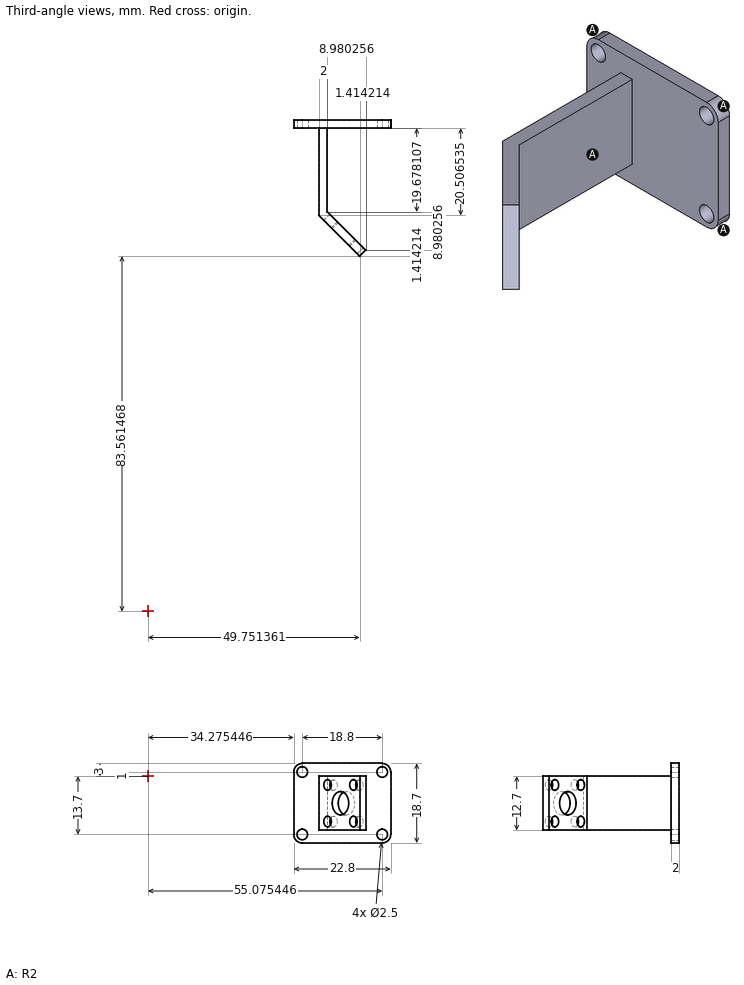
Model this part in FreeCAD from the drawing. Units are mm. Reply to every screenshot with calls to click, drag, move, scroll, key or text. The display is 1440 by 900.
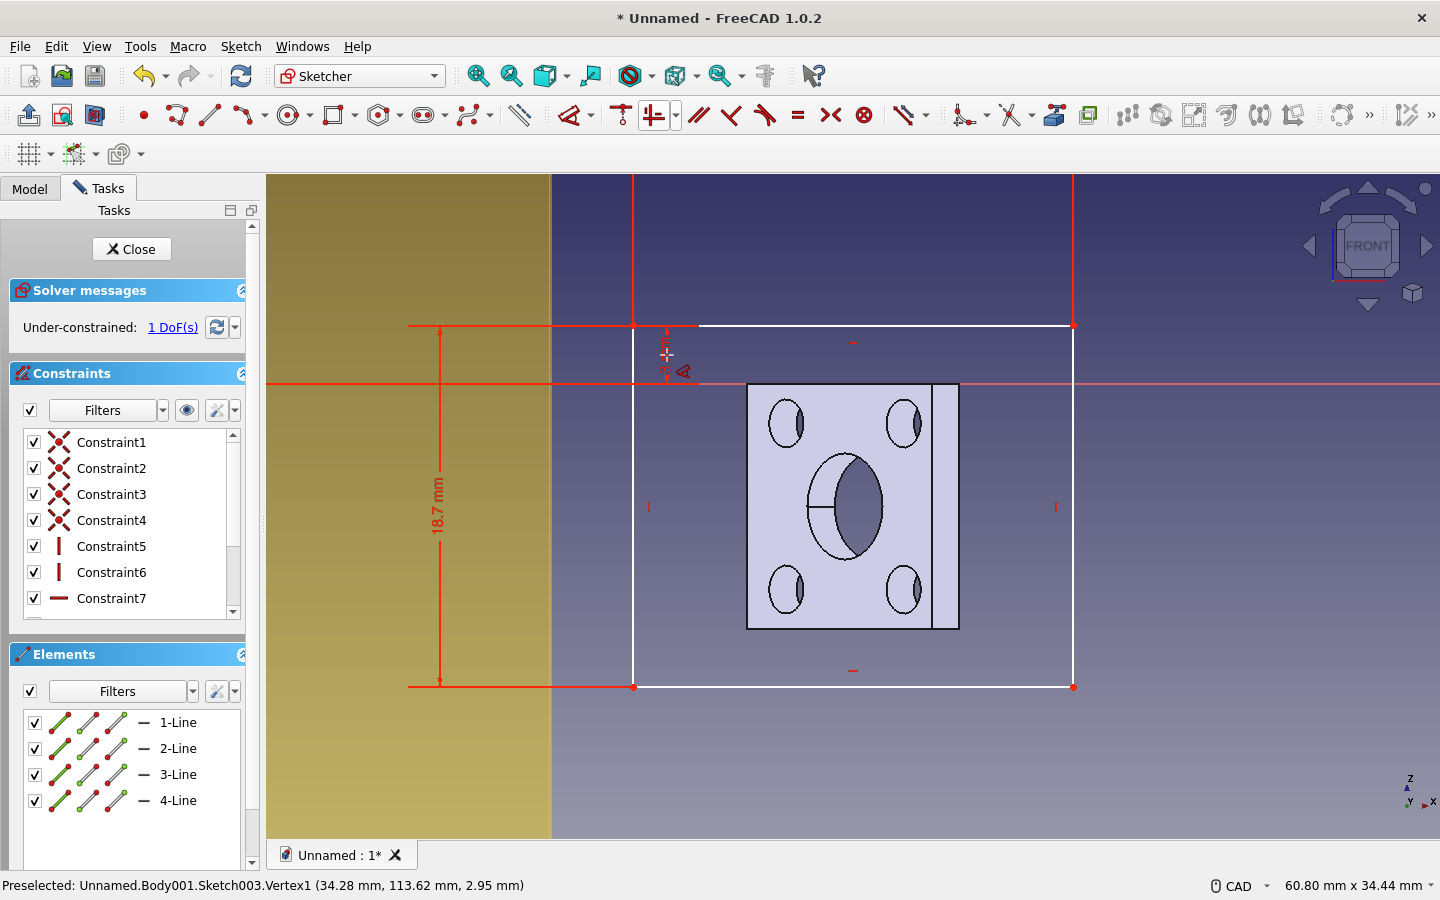
click(633, 326)
click(463, 292)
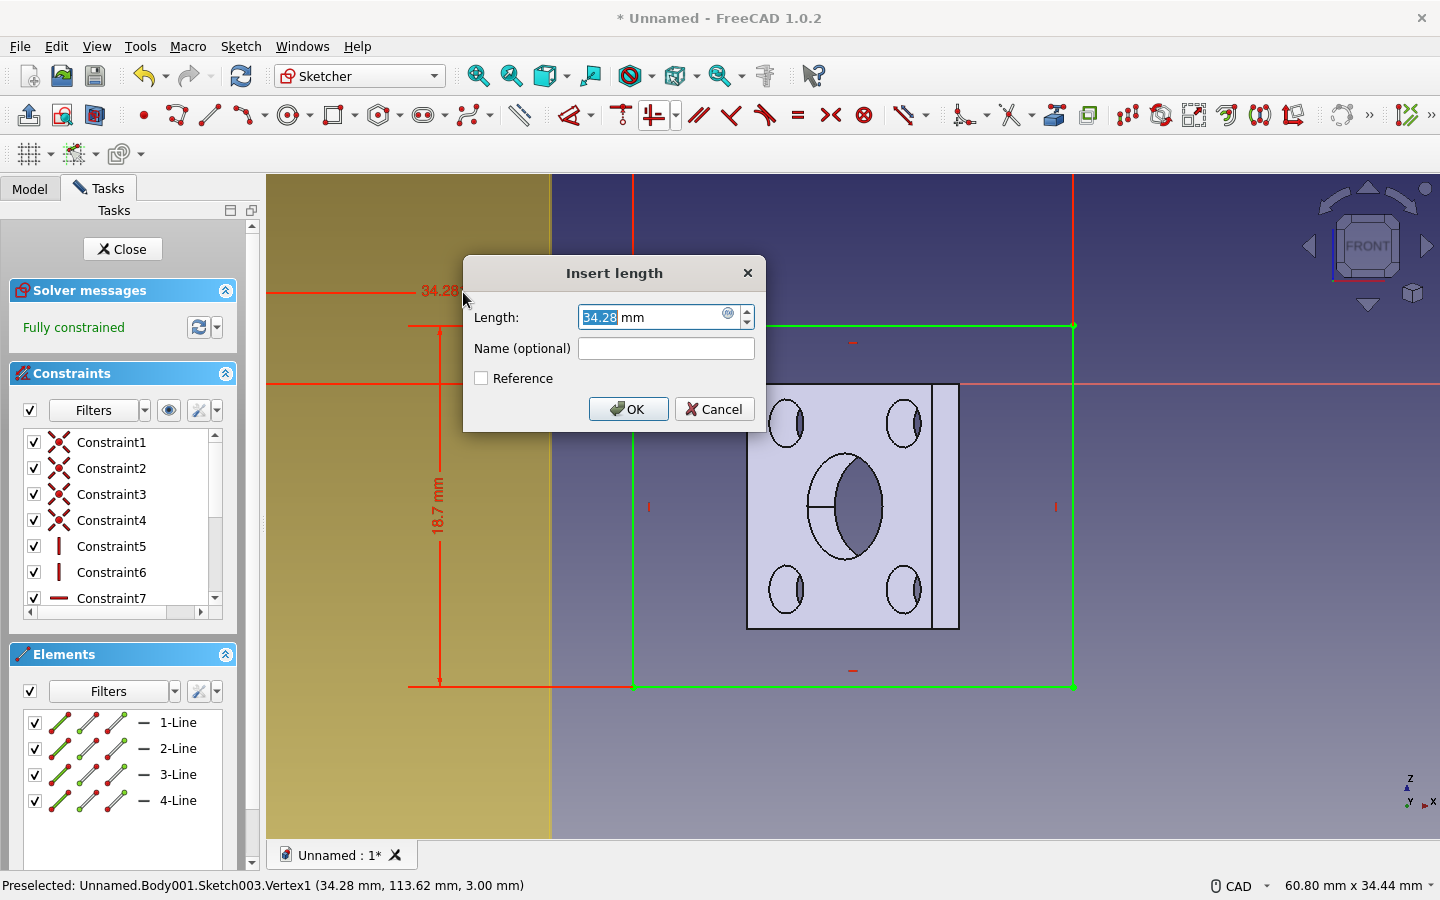
text(34.275446)
key(Return)
key(Escape)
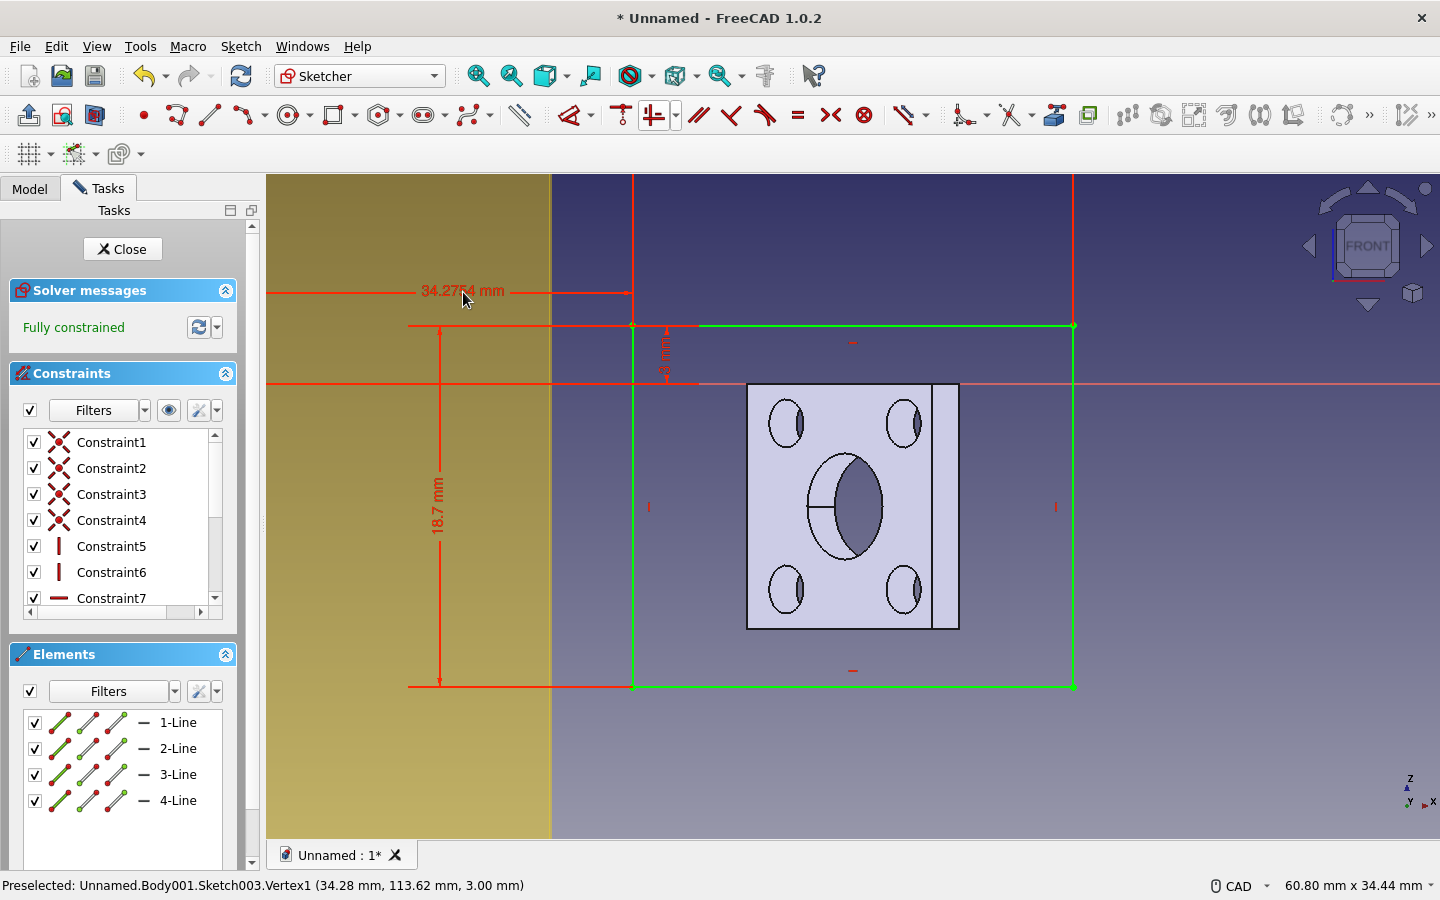
click(123, 249)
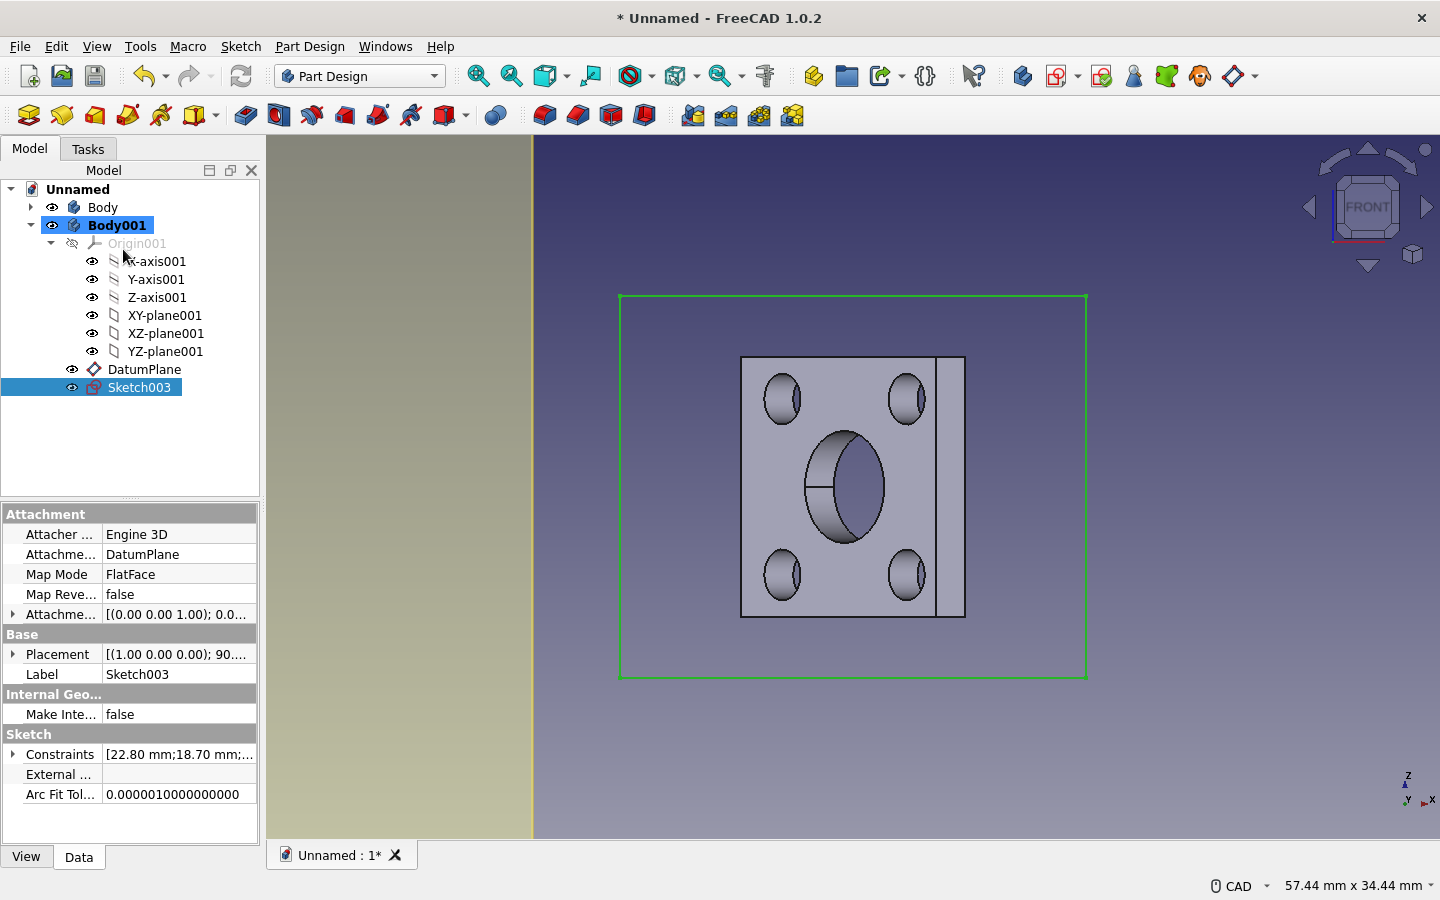
click(29, 116)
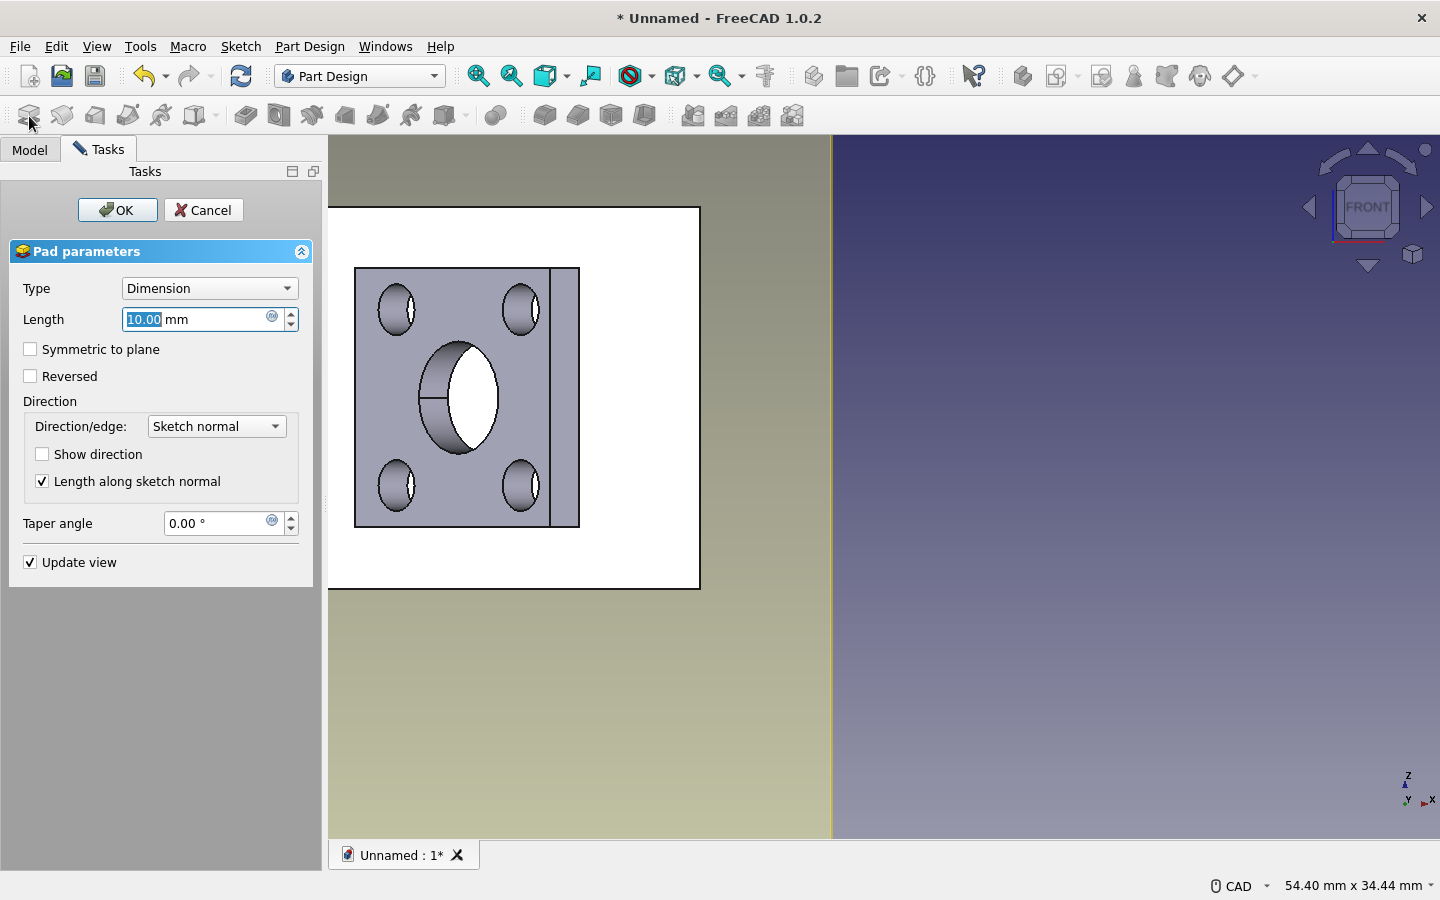
text(2)
key(Tab)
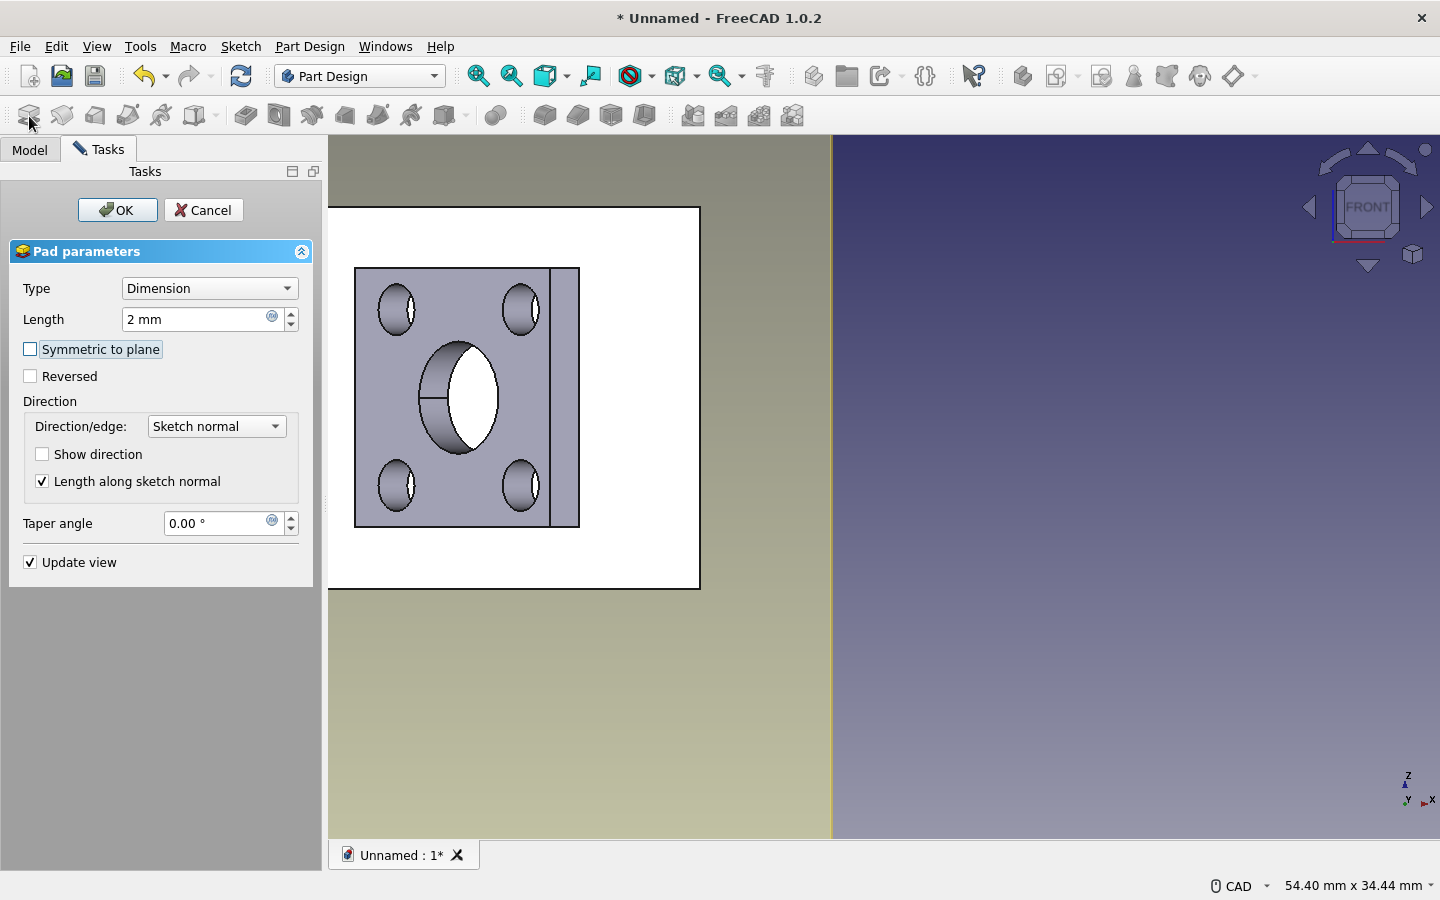
click(31, 376)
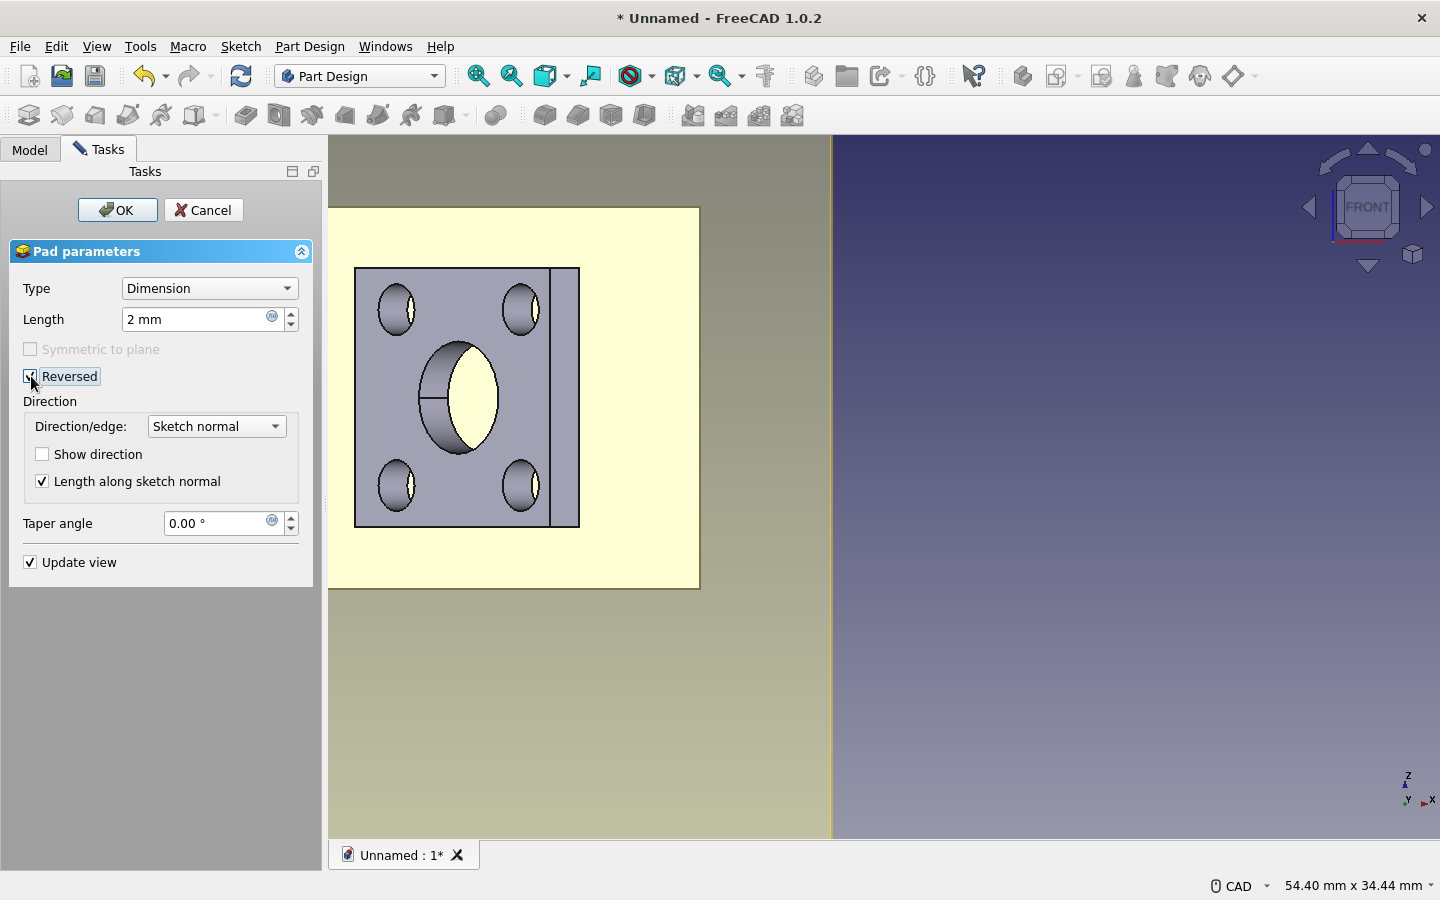
click(118, 210)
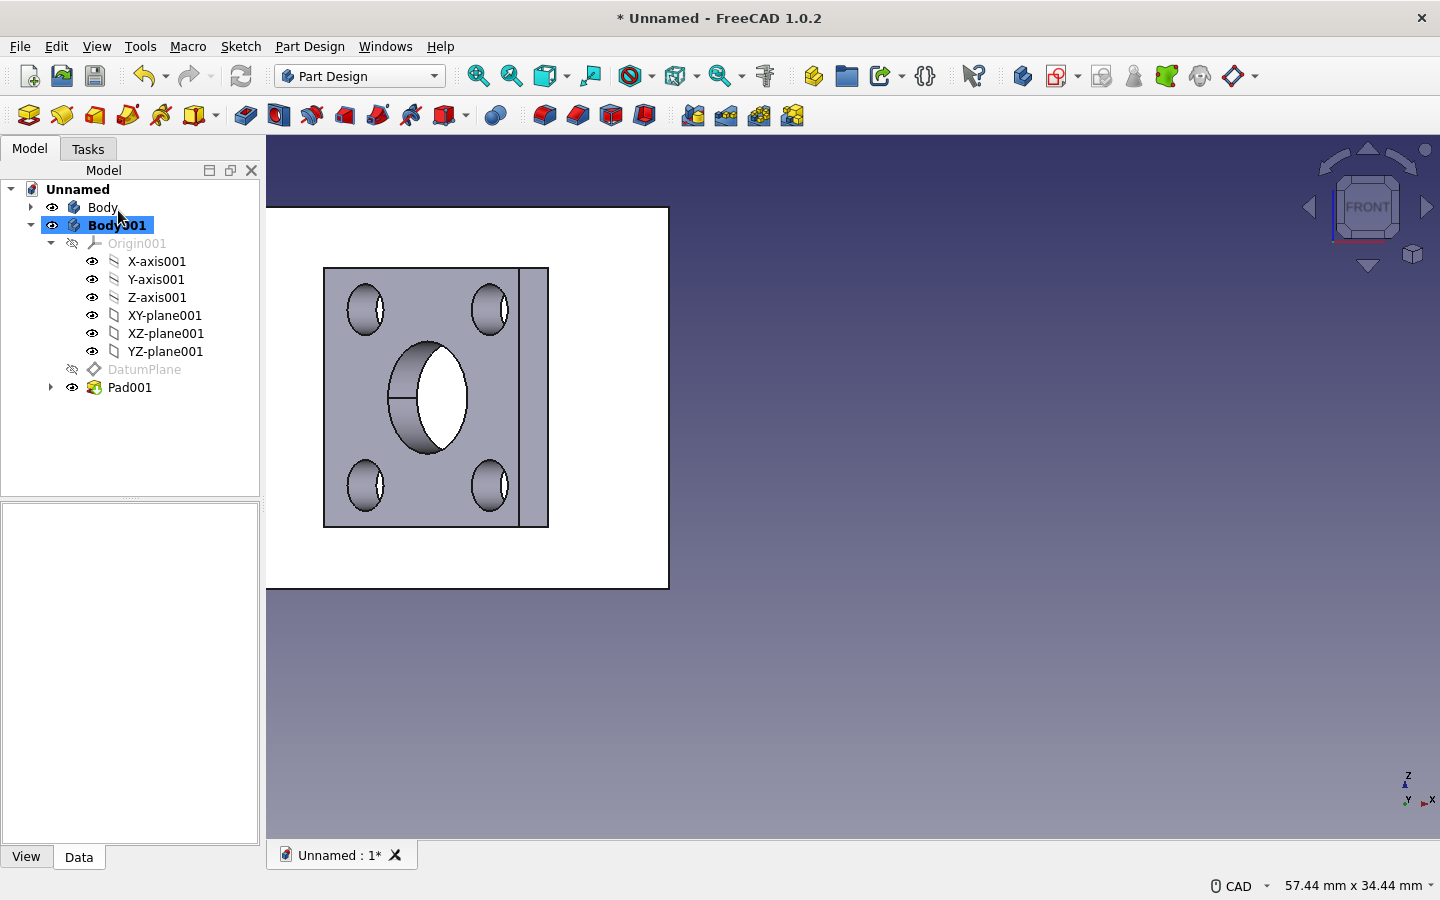
click(479, 76)